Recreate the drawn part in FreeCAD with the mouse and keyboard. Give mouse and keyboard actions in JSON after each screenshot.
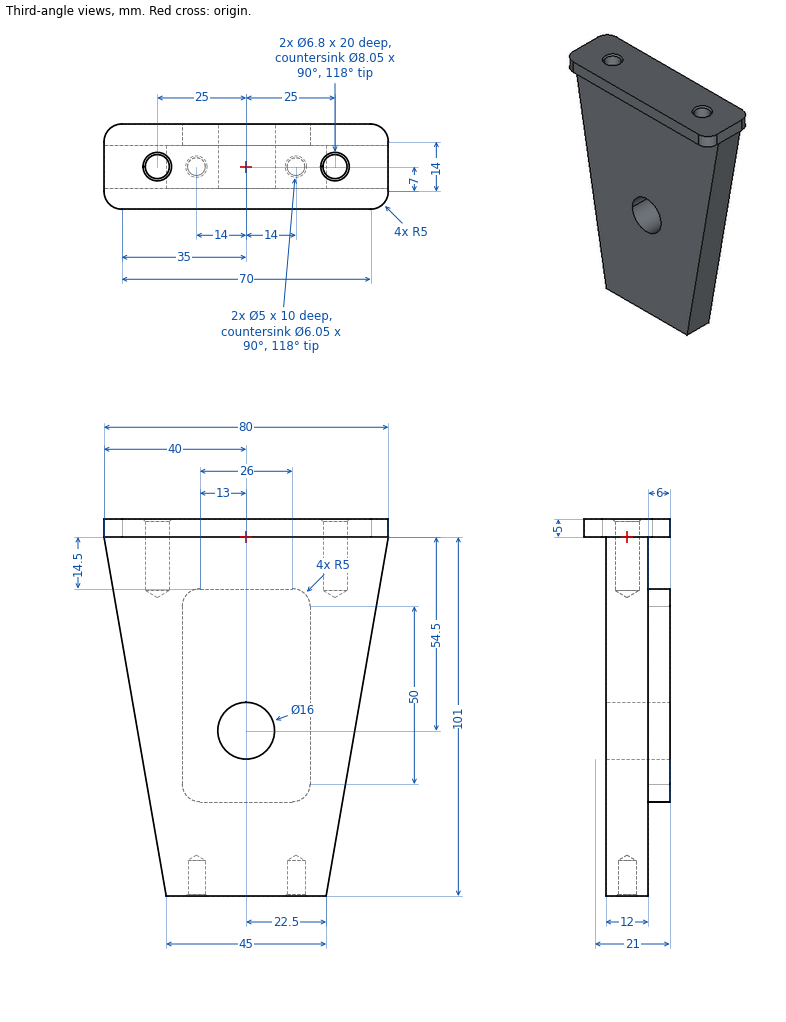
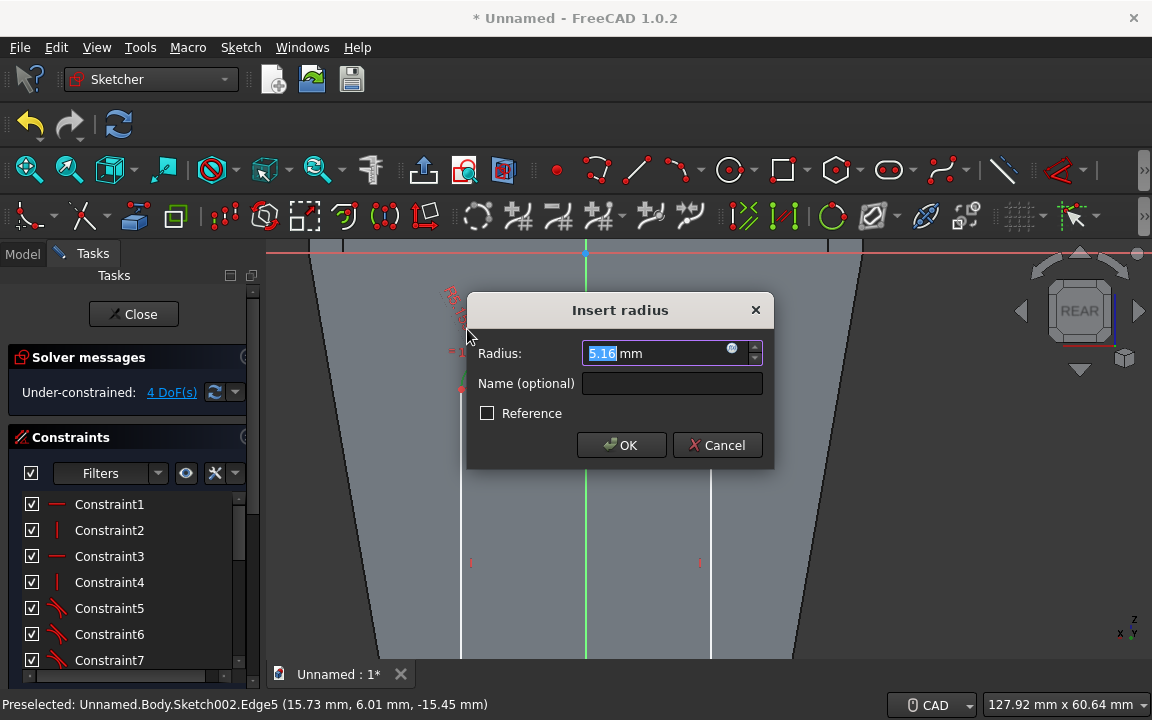
{"action": "type", "text": "5"}
{"action": "key", "text": "Return"}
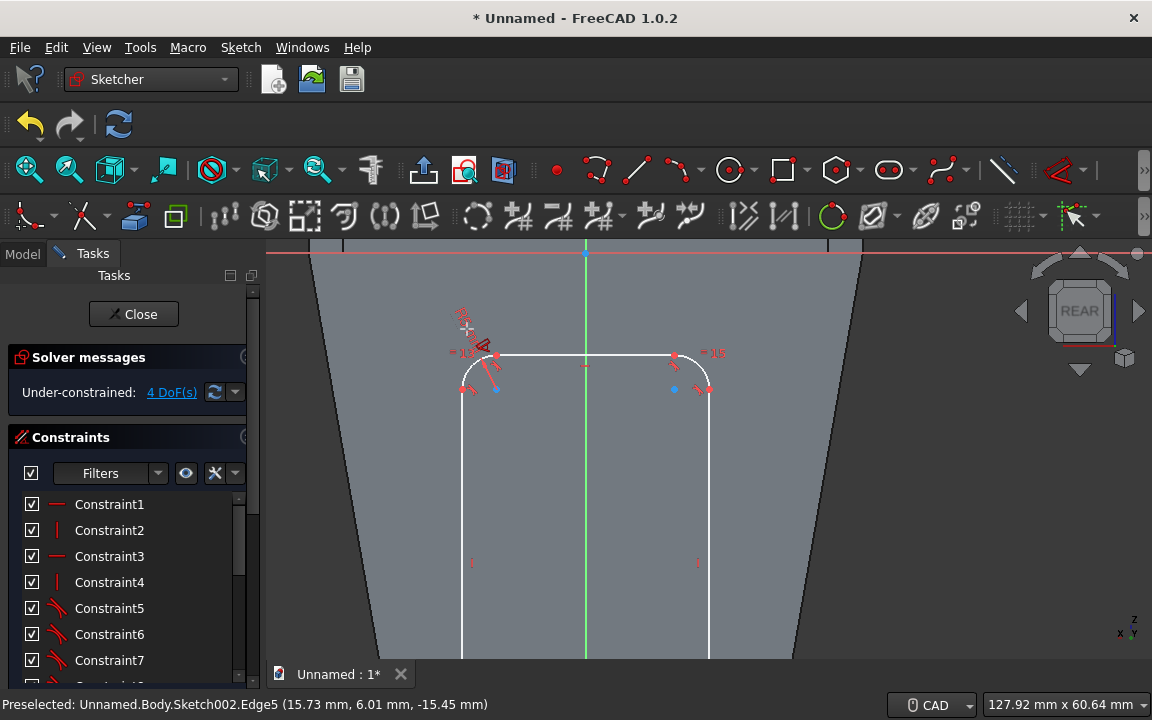
{"action": "left_click", "coordinate": [621, 355]}
{"action": "left_click", "coordinate": [545, 321]}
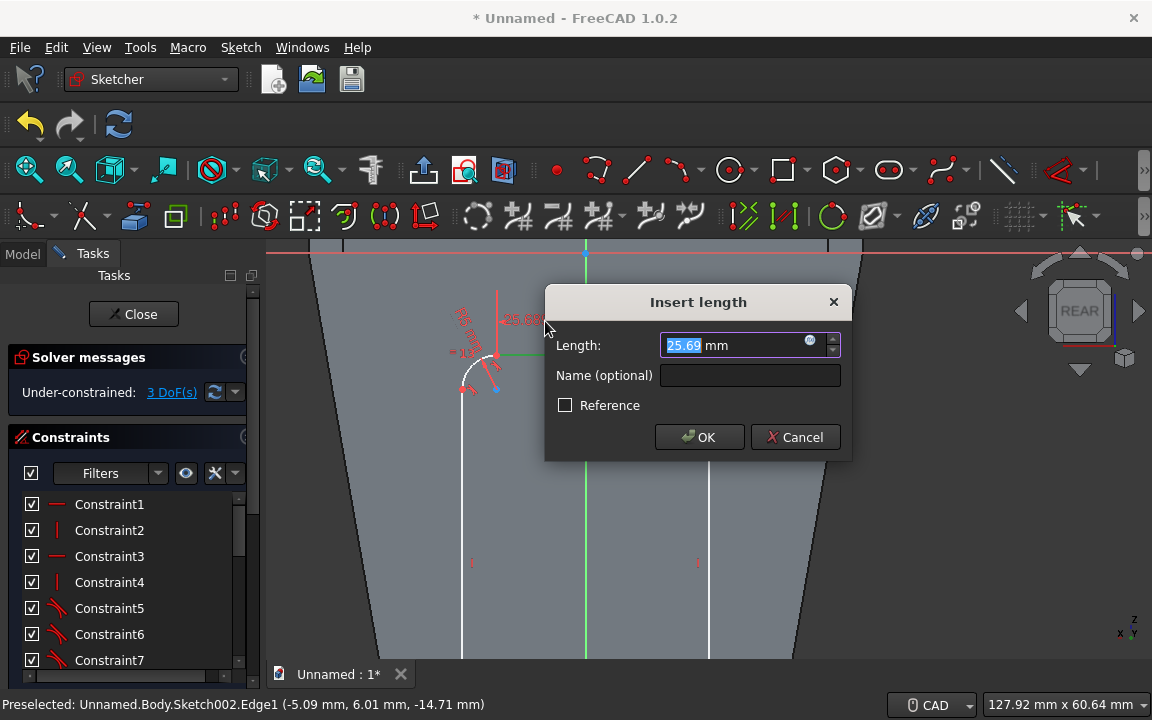
{"action": "type", "text": "26"}
{"action": "key", "text": "Return"}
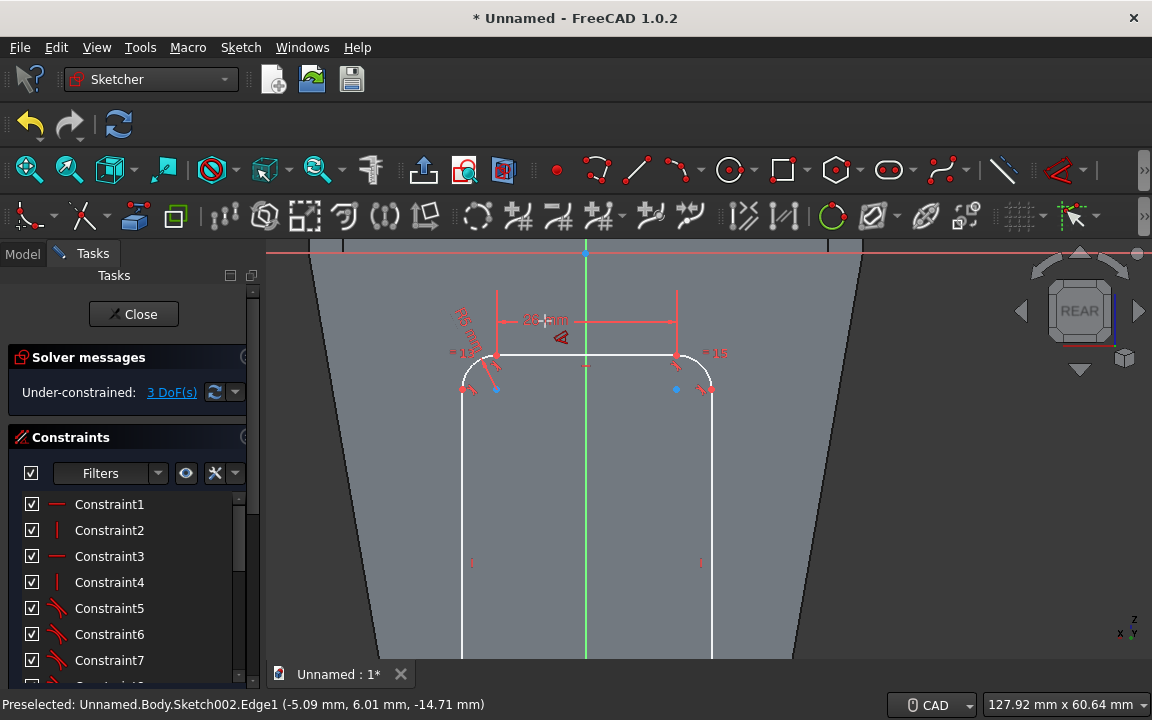
{"action": "left_click", "coordinate": [462, 494]}
{"action": "left_click", "coordinate": [428, 510]}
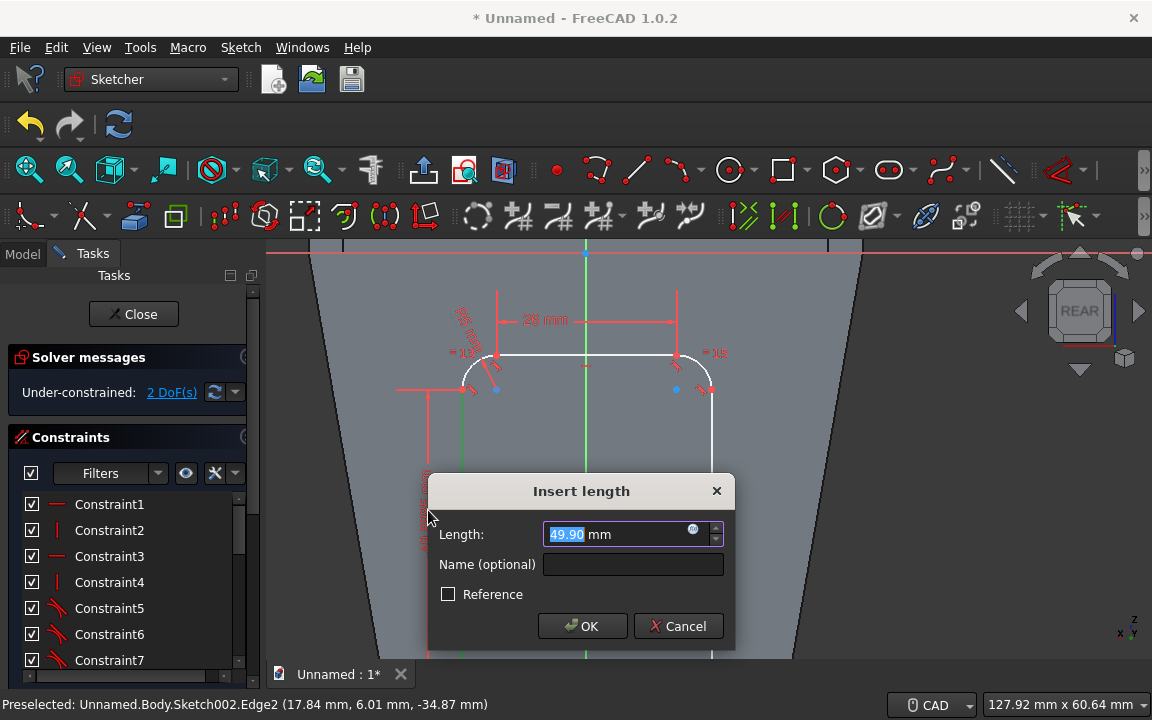
{"action": "type", "text": "50"}
{"action": "key", "text": "Return"}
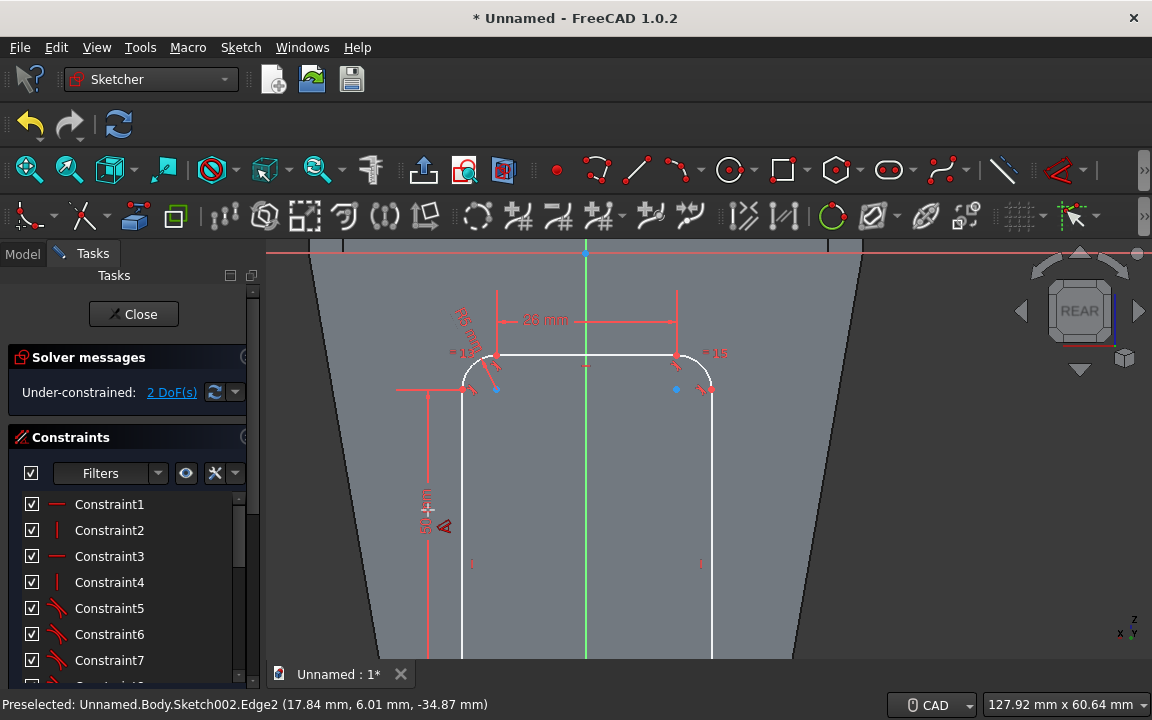
{"action": "left_click", "coordinate": [677, 355]}
{"action": "left_click", "coordinate": [631, 389]}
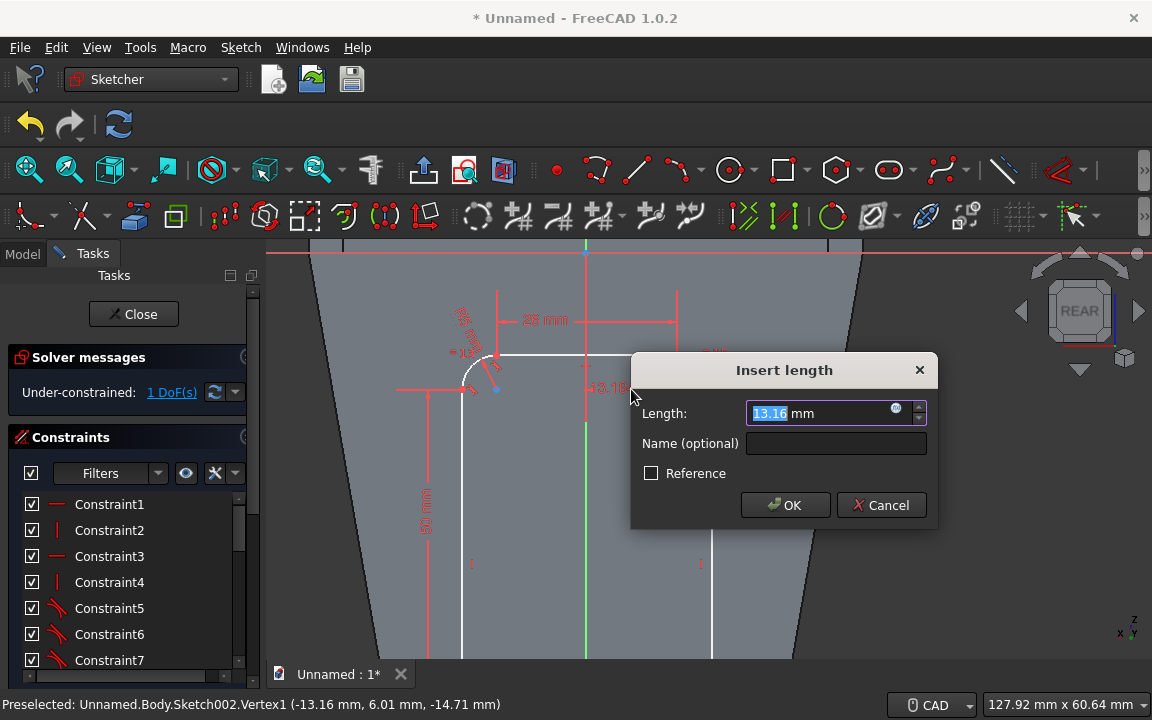
{"action": "type", "text": "13"}
{"action": "key", "text": "Return"}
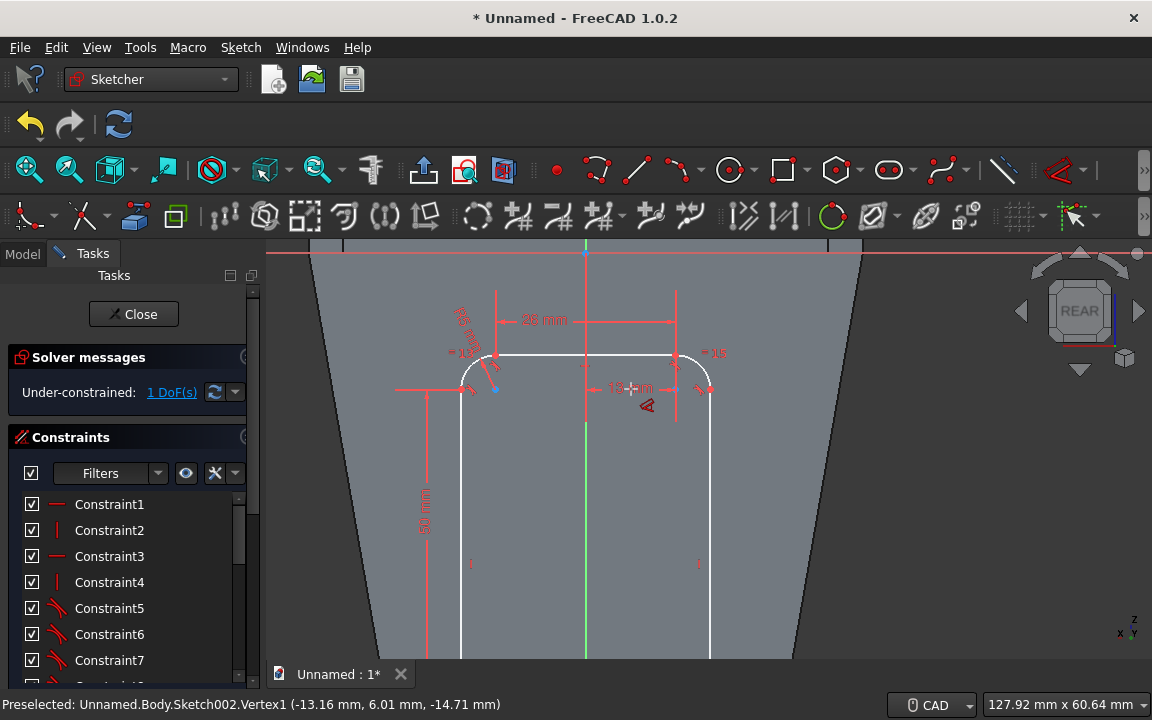
{"action": "left_click", "coordinate": [676, 355]}
{"action": "left_click", "coordinate": [710, 311]}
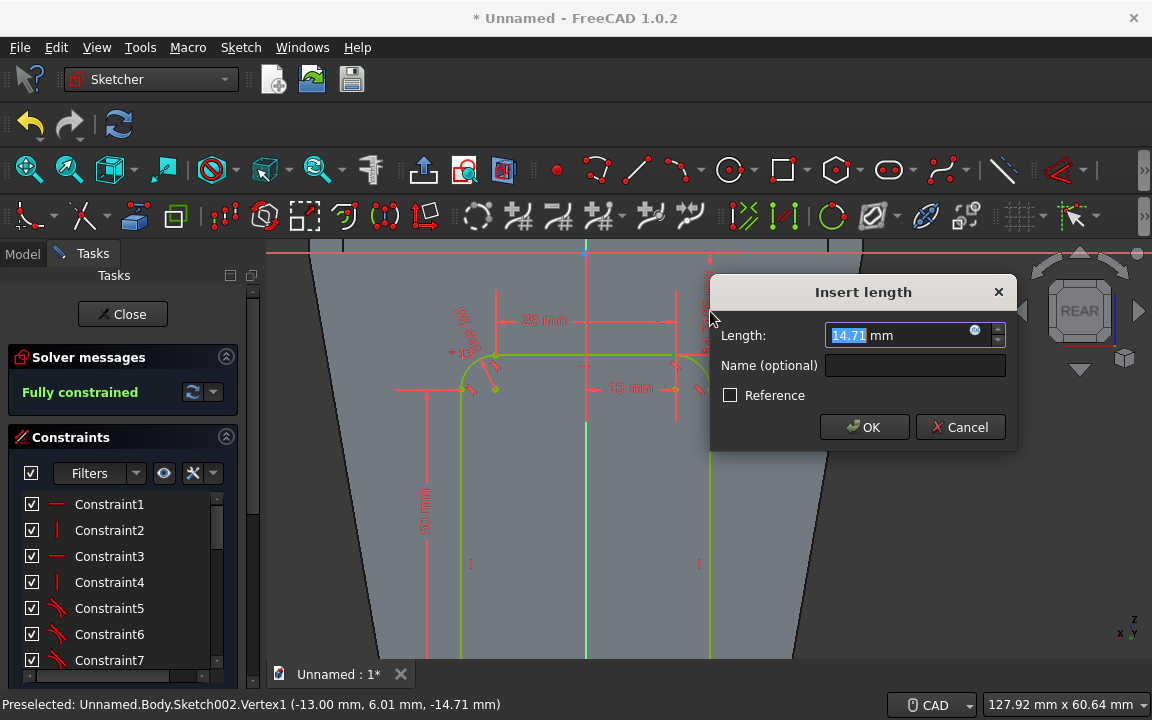
{"action": "type", "text": "14.5"}
{"action": "key", "text": "Return"}
{"action": "key", "text": "Escape"}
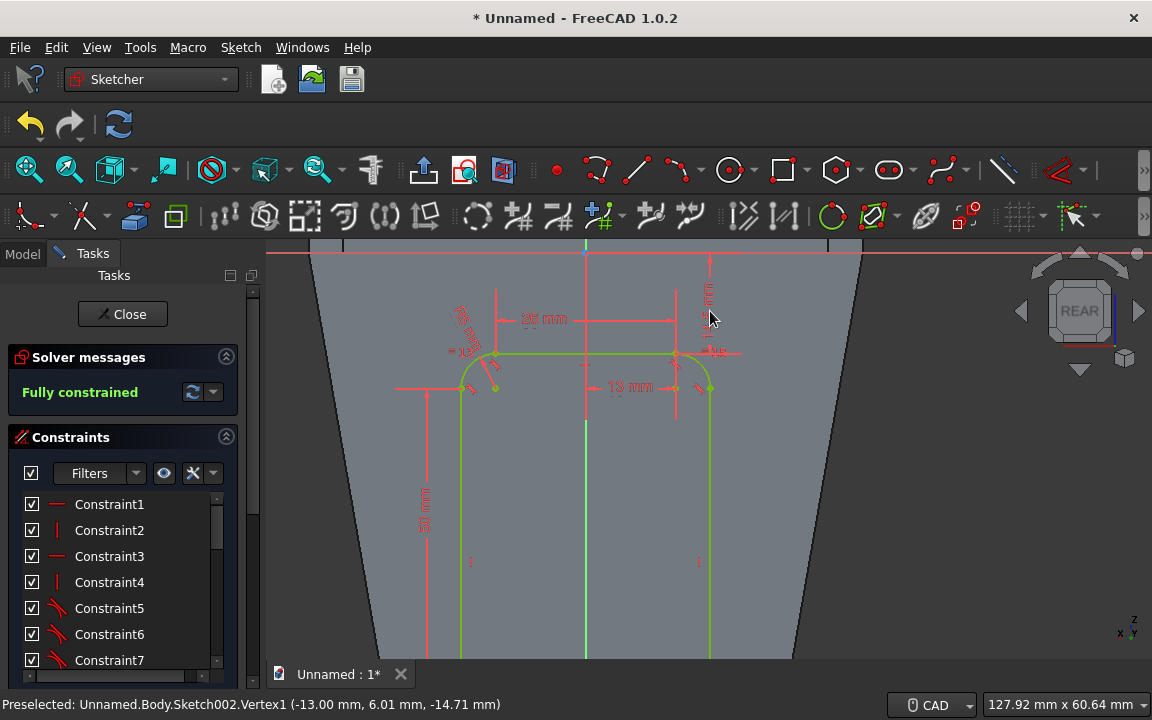
{"action": "left_click", "coordinate": [123, 314]}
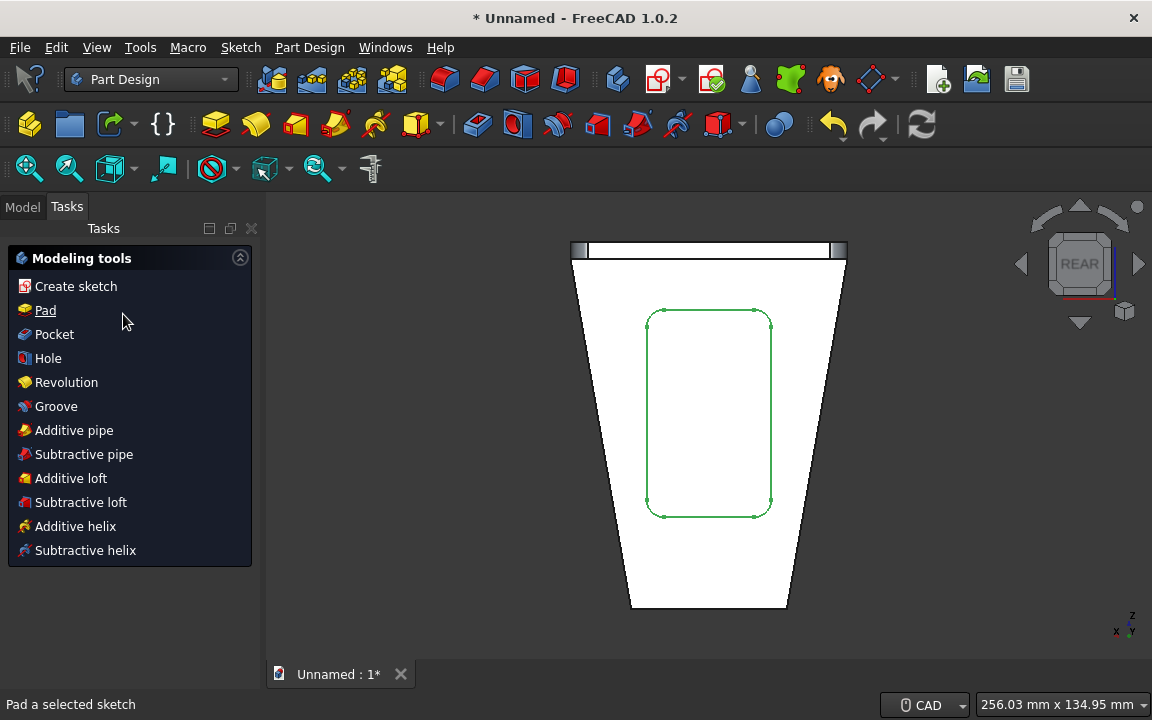
{"action": "left_click", "coordinate": [216, 124]}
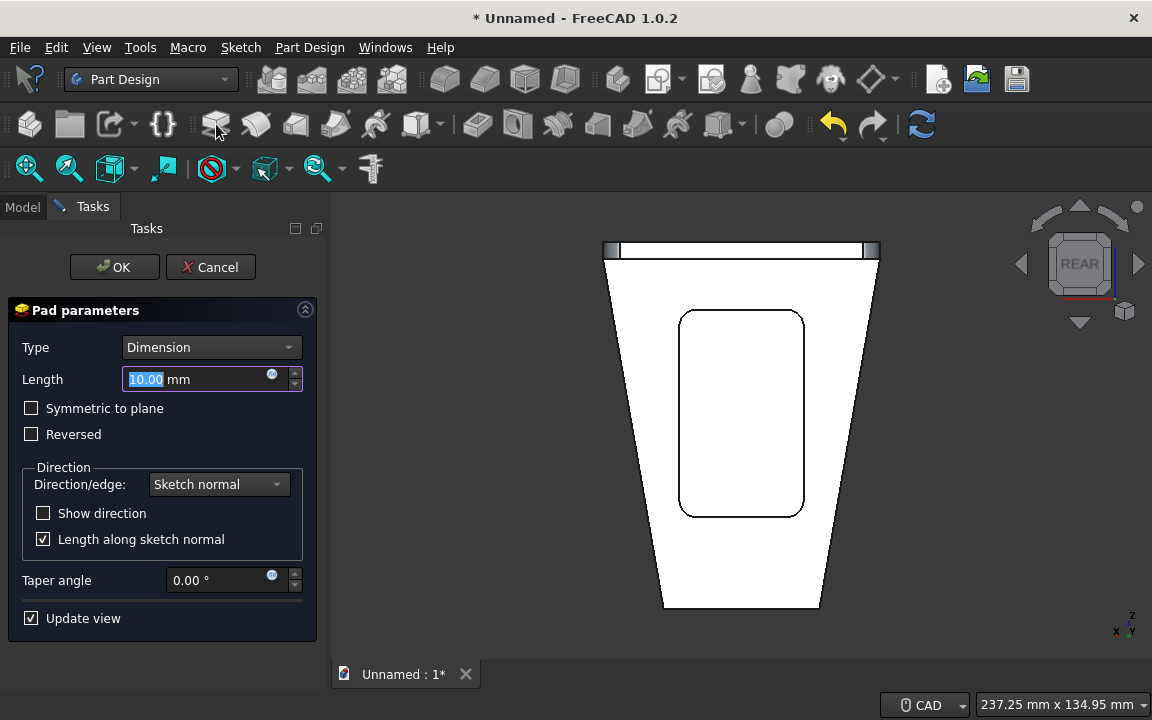
{"action": "type", "text": "6"}
{"action": "key", "text": "Tab"}